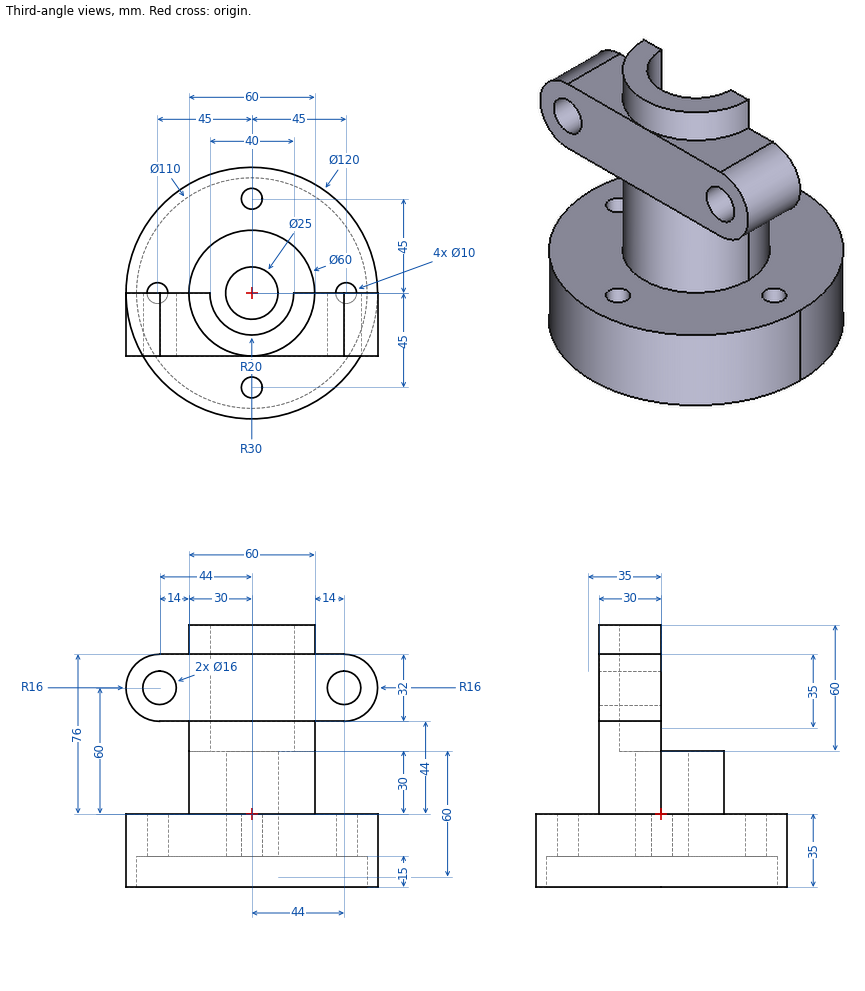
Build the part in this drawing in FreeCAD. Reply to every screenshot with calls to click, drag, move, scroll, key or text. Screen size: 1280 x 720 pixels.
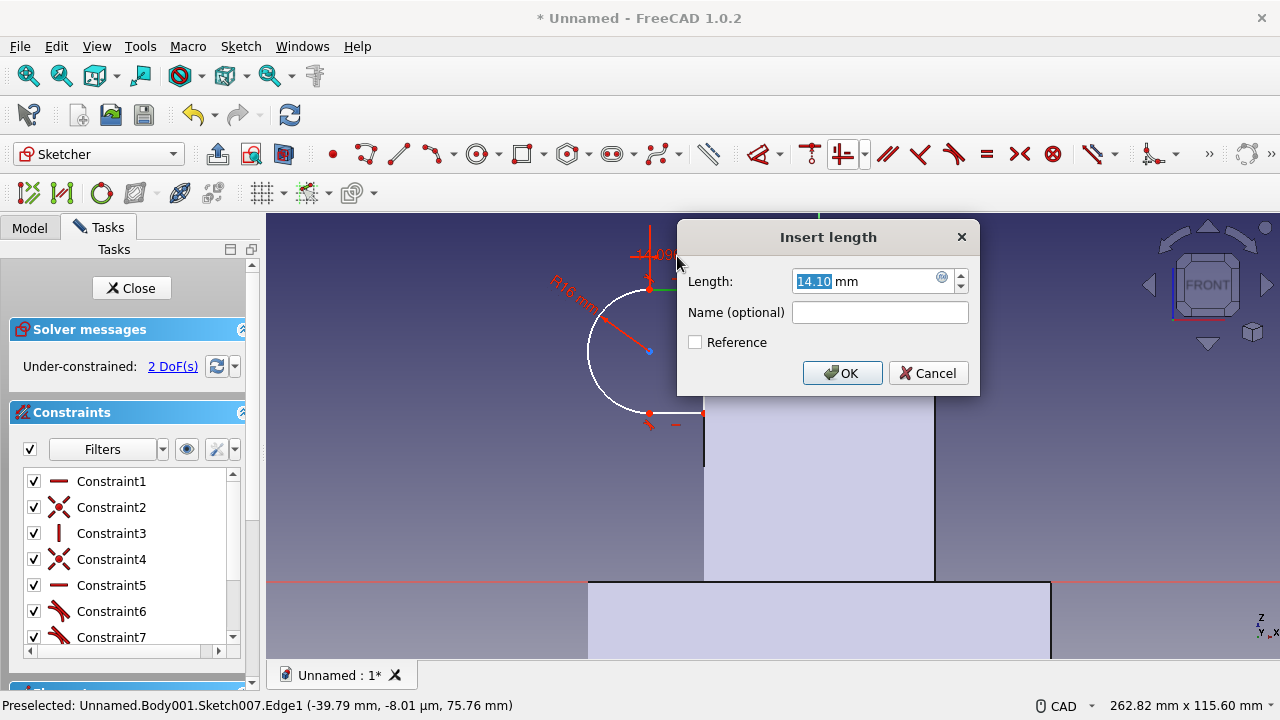
text(14)
key(Return)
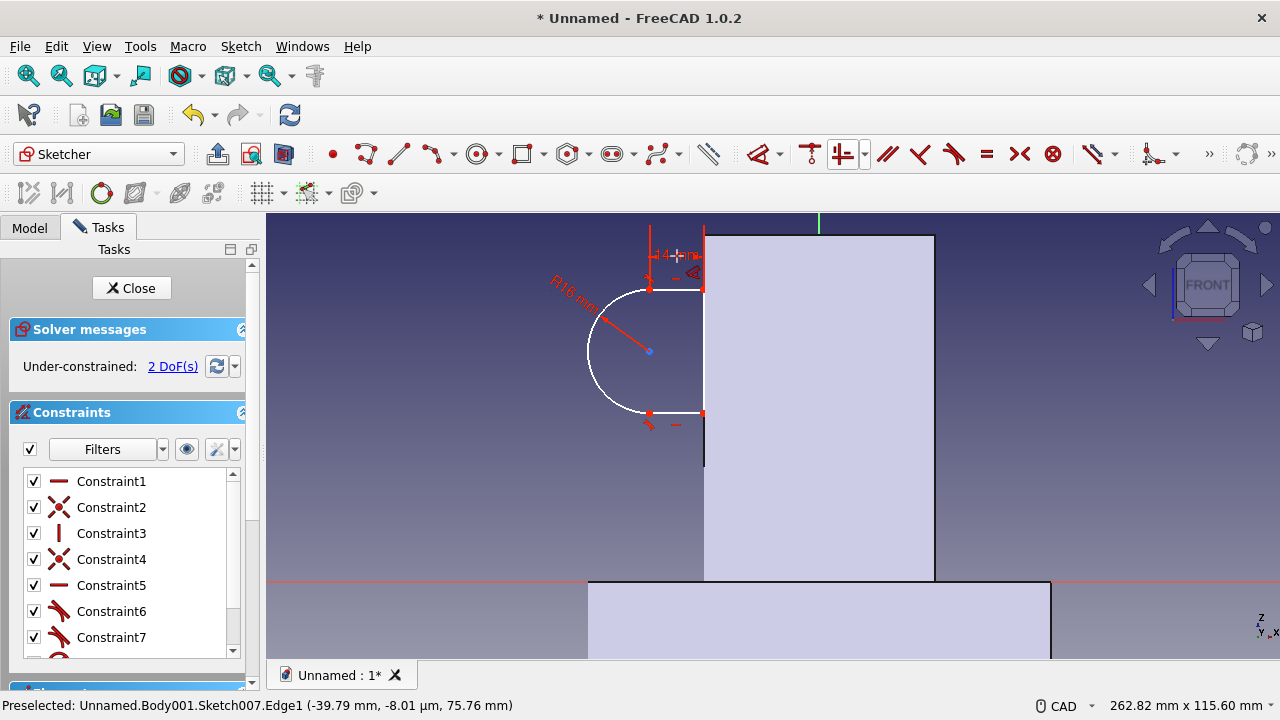
click(650, 290)
click(735, 616)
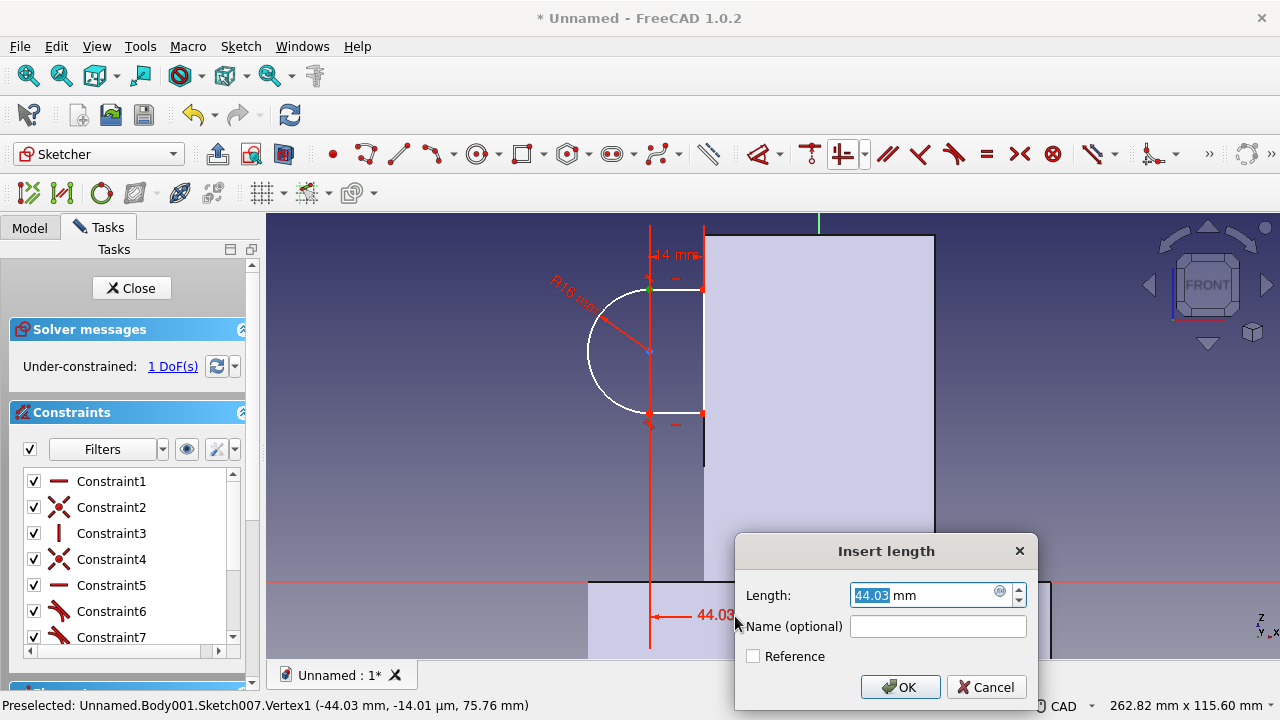
text(44)
key(Return)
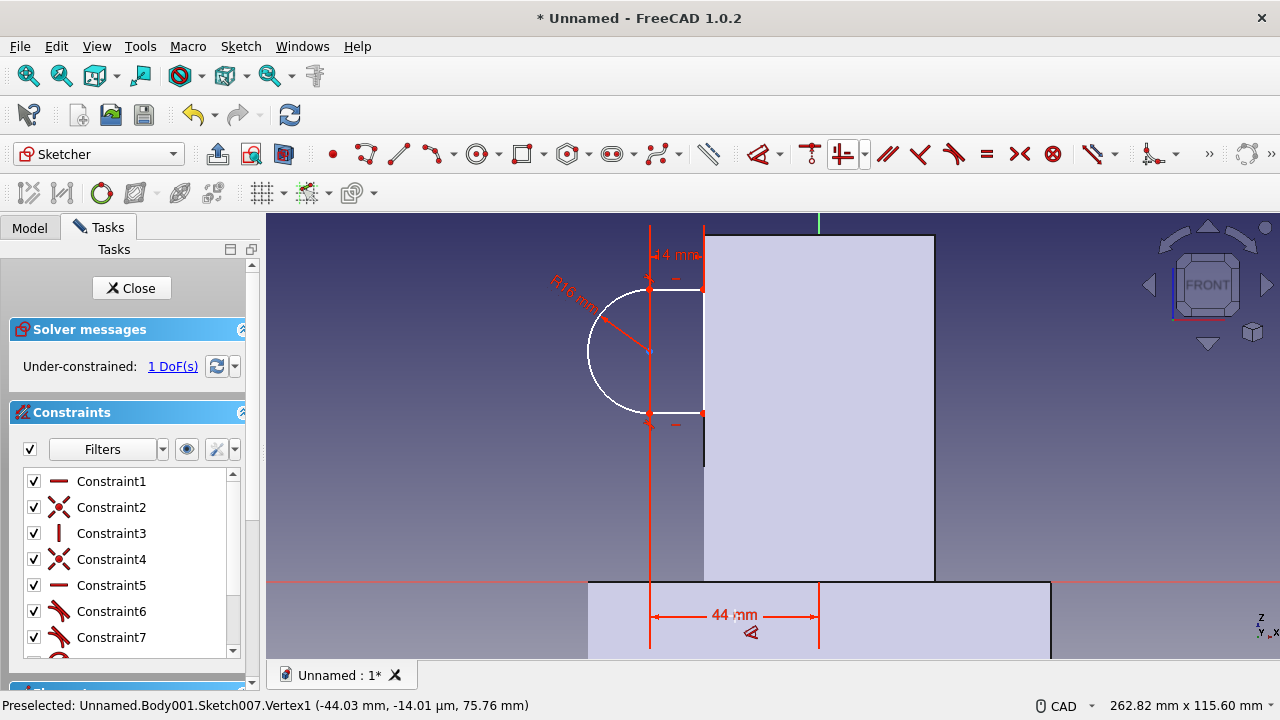
click(650, 290)
click(853, 436)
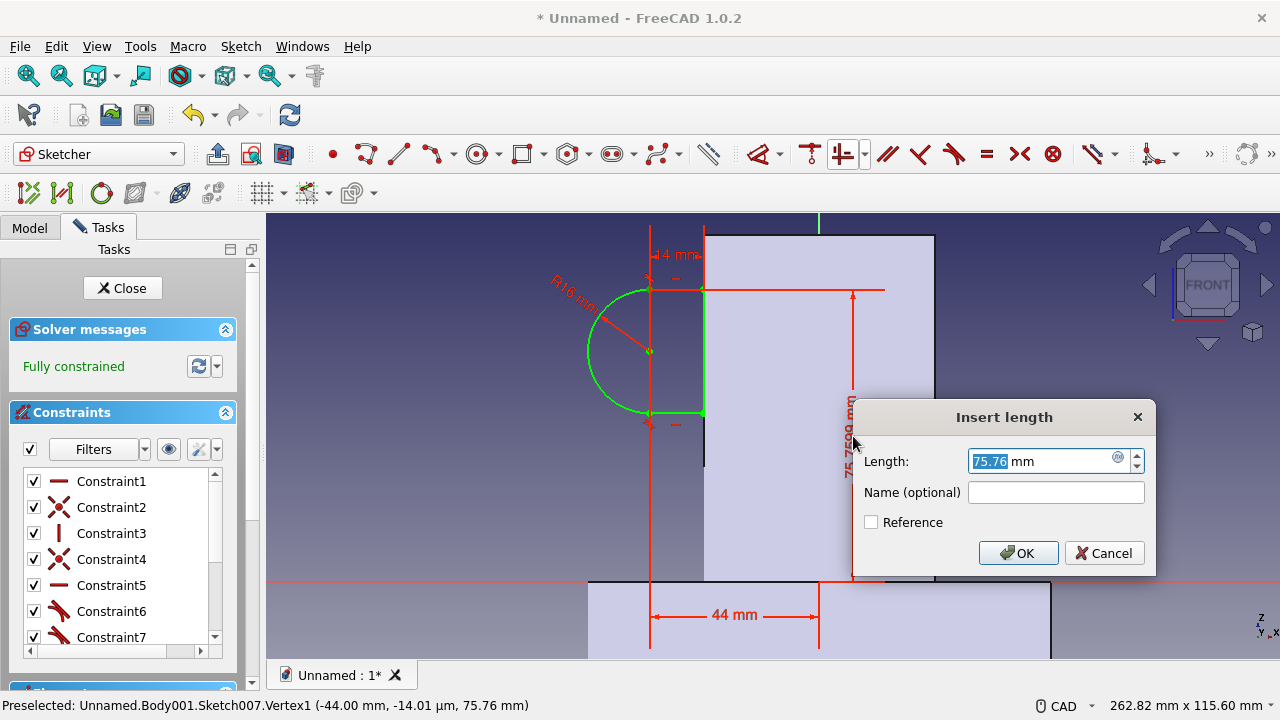
text(76)
key(Return)
key(Escape)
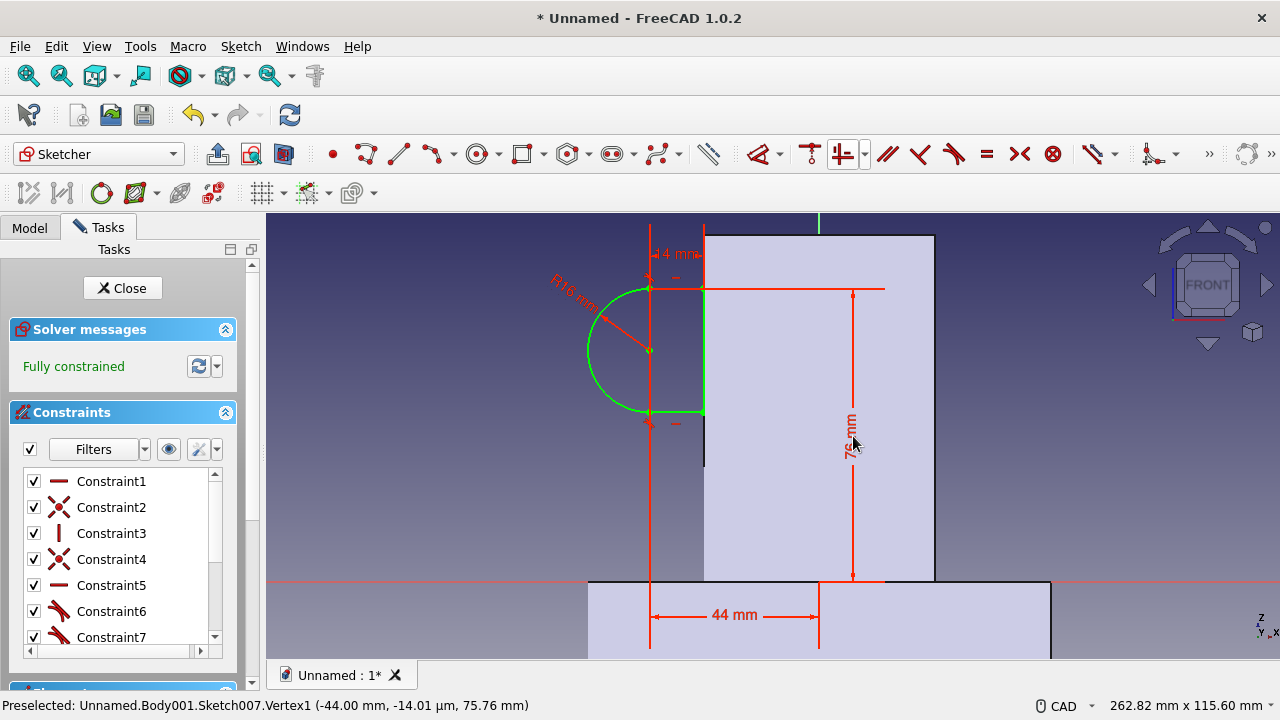
click(123, 288)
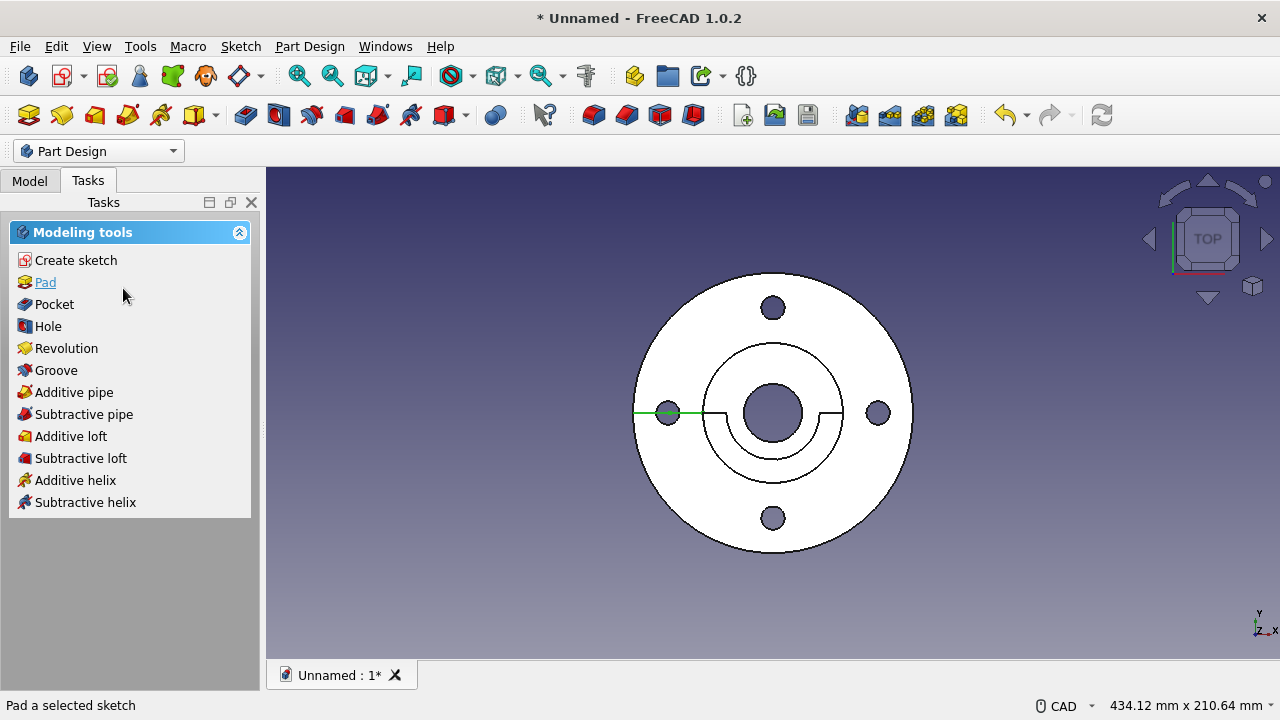
click(29, 116)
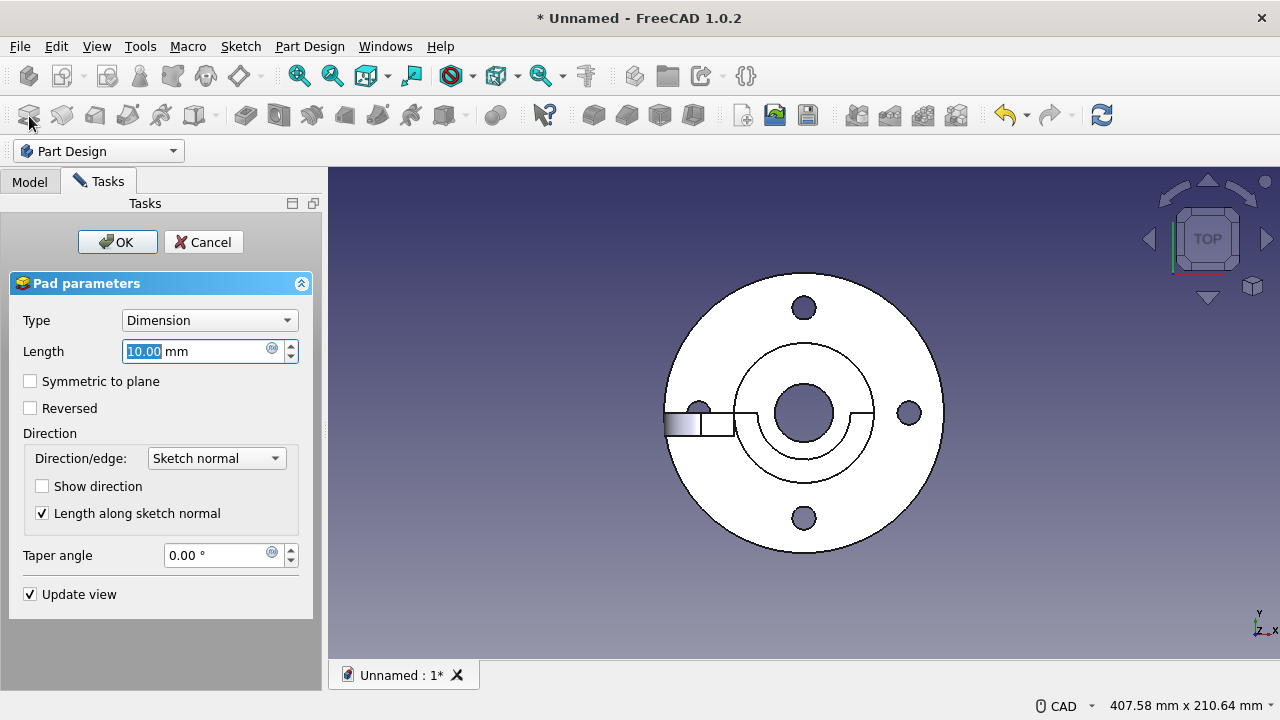
text(30)
key(Tab)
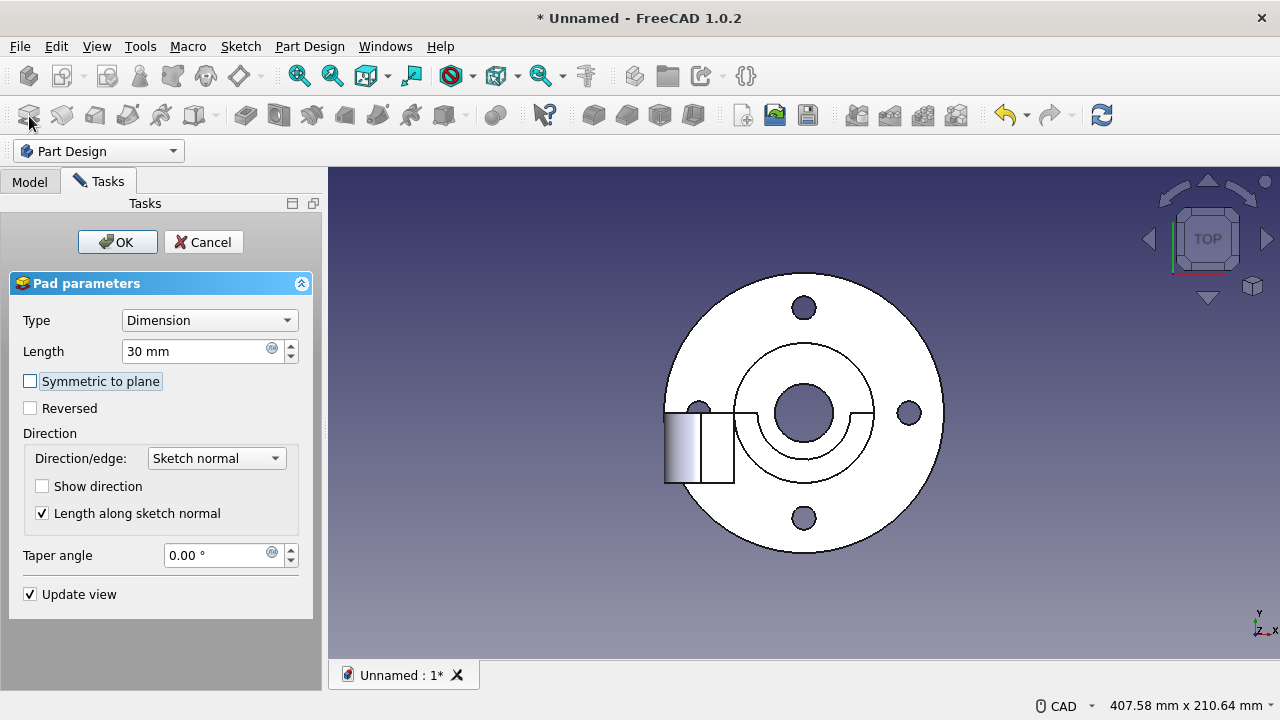
click(118, 242)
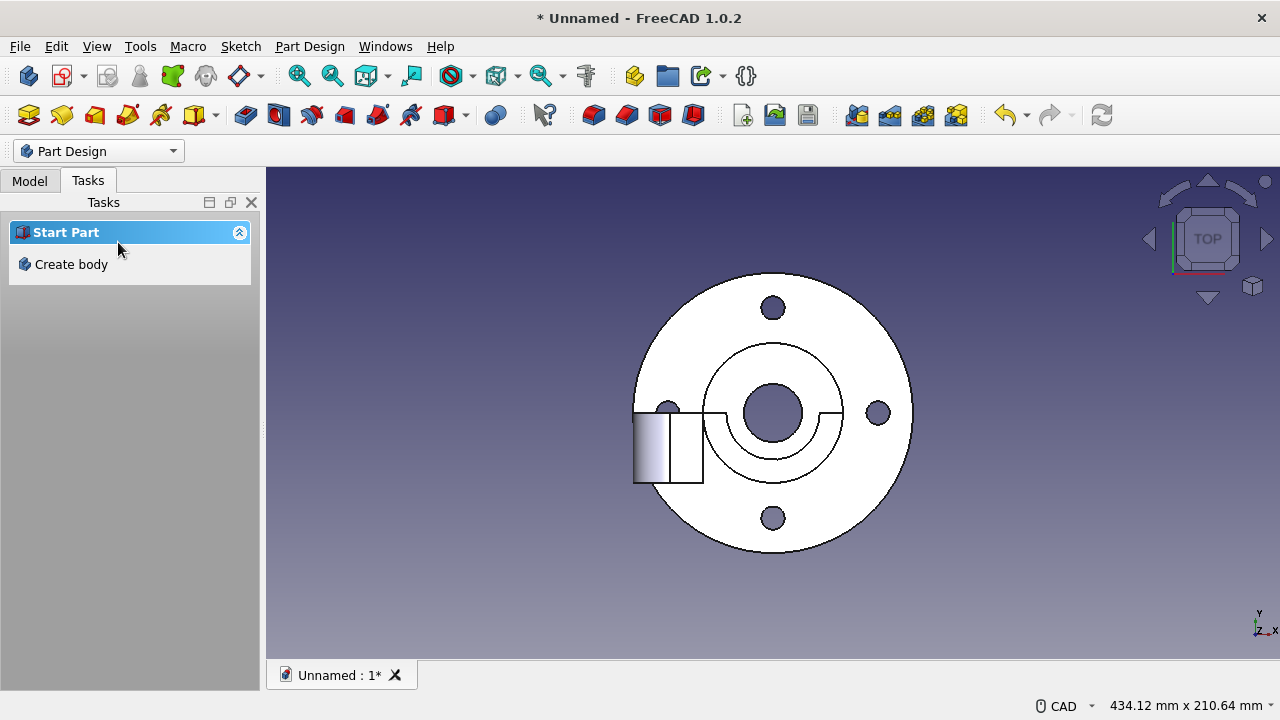
click(300, 76)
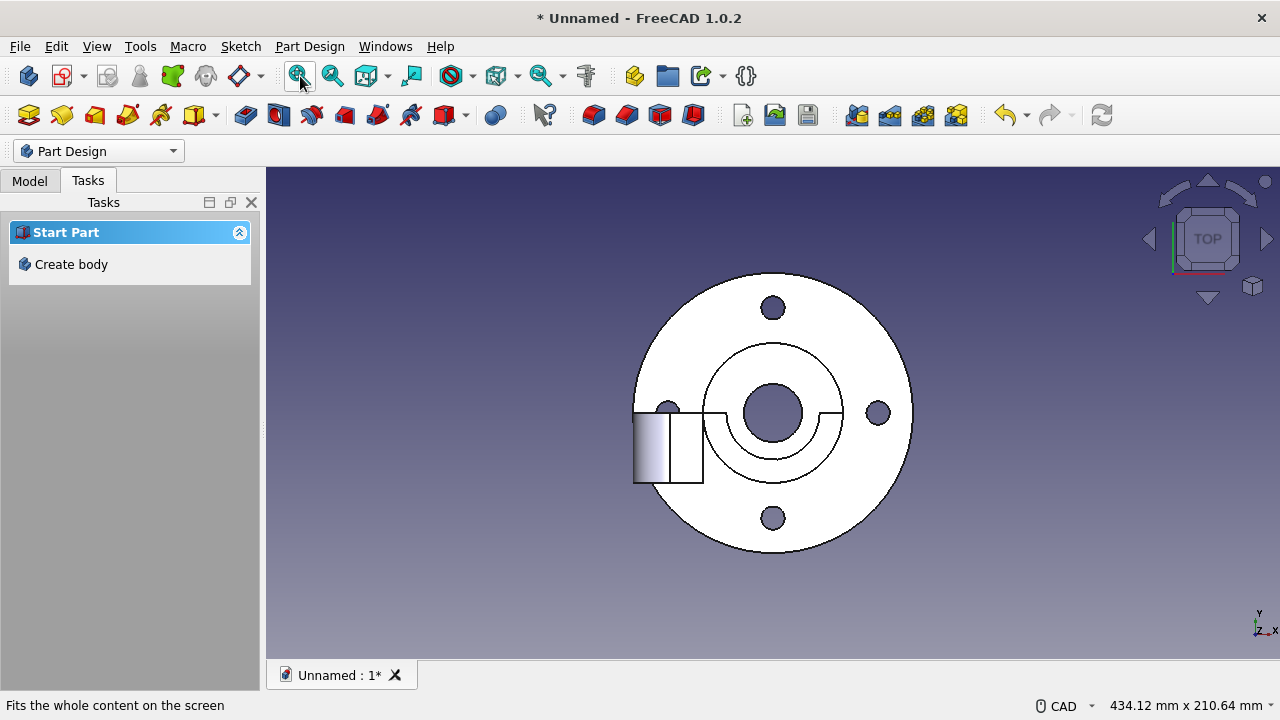
click(29, 76)